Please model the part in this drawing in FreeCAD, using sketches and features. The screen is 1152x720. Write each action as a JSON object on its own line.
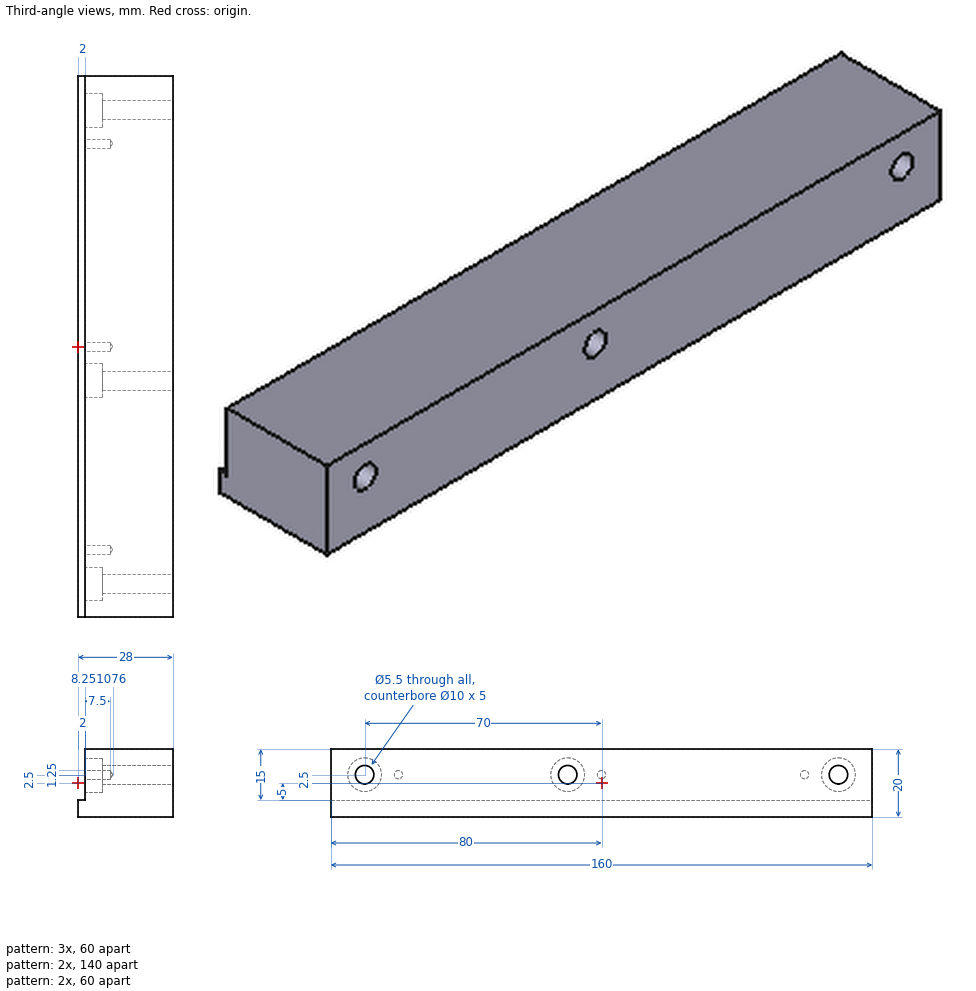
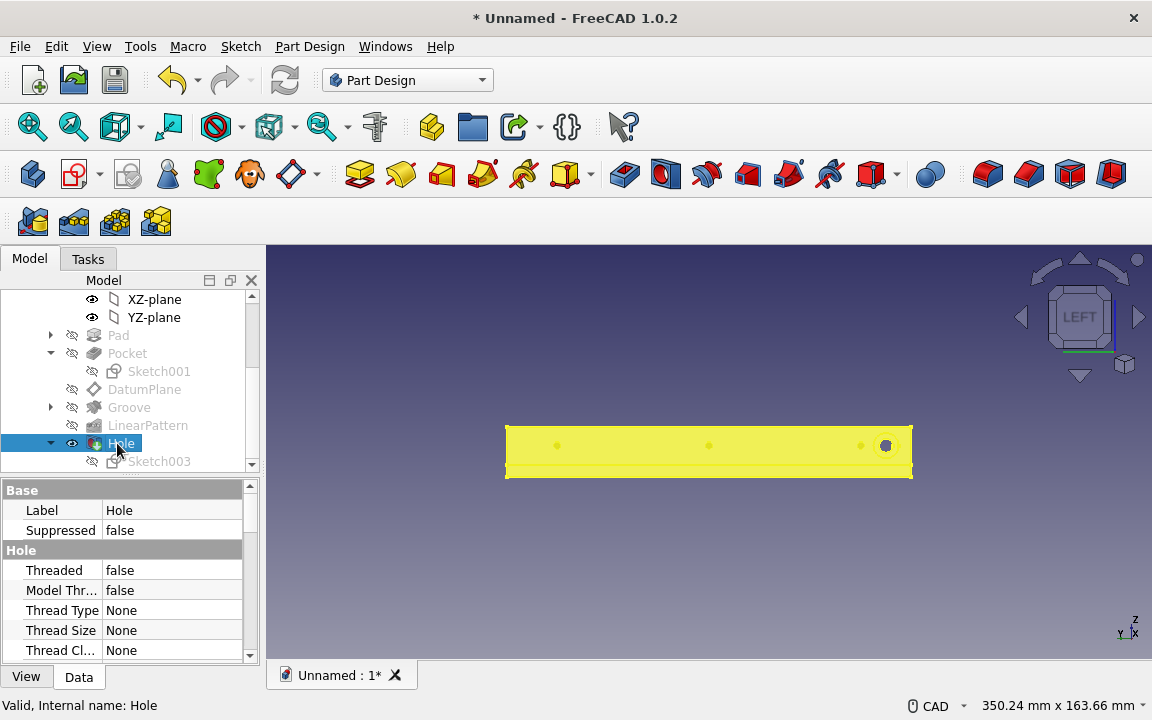
{"action": "left_click", "coordinate": [74, 222]}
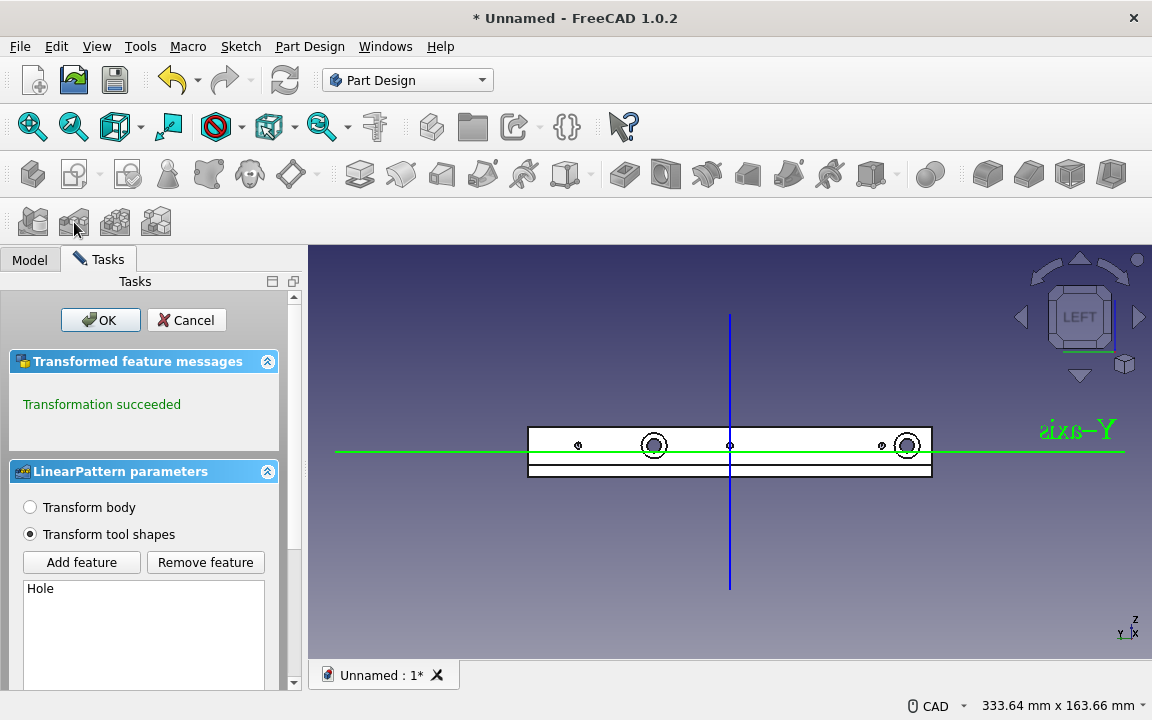
{"action": "scroll", "coordinate": [294, 490], "scroll_direction": "down", "scroll_amount": 2}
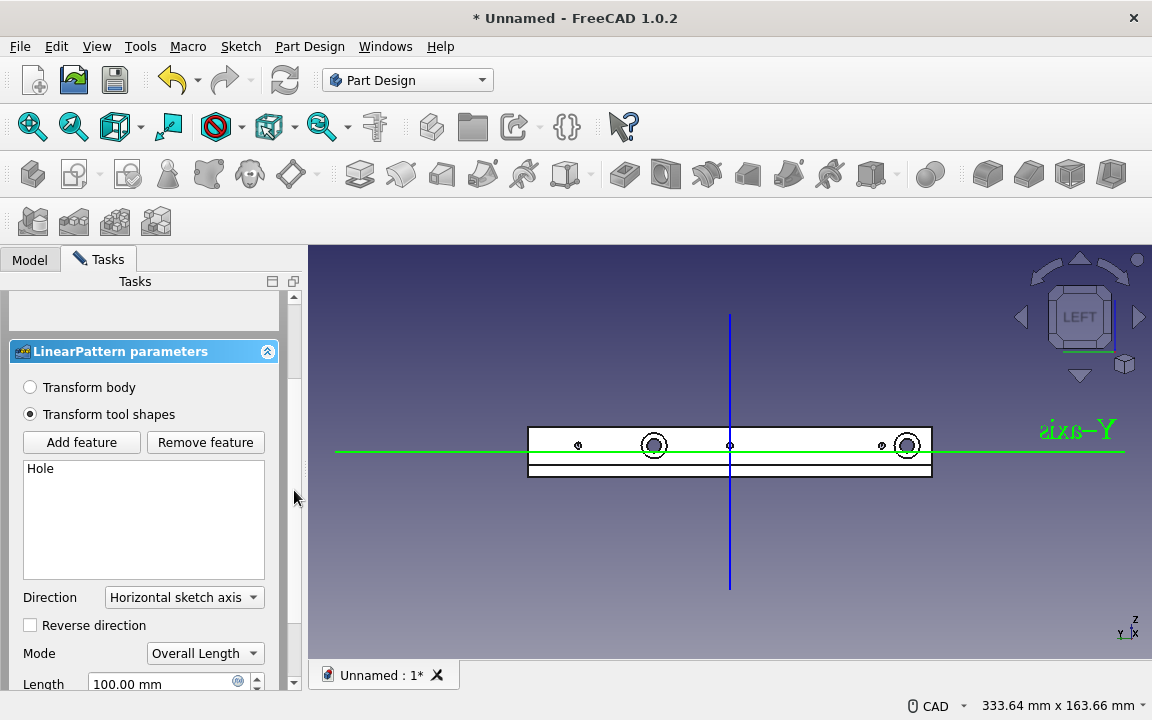
{"action": "left_click", "coordinate": [185, 598]}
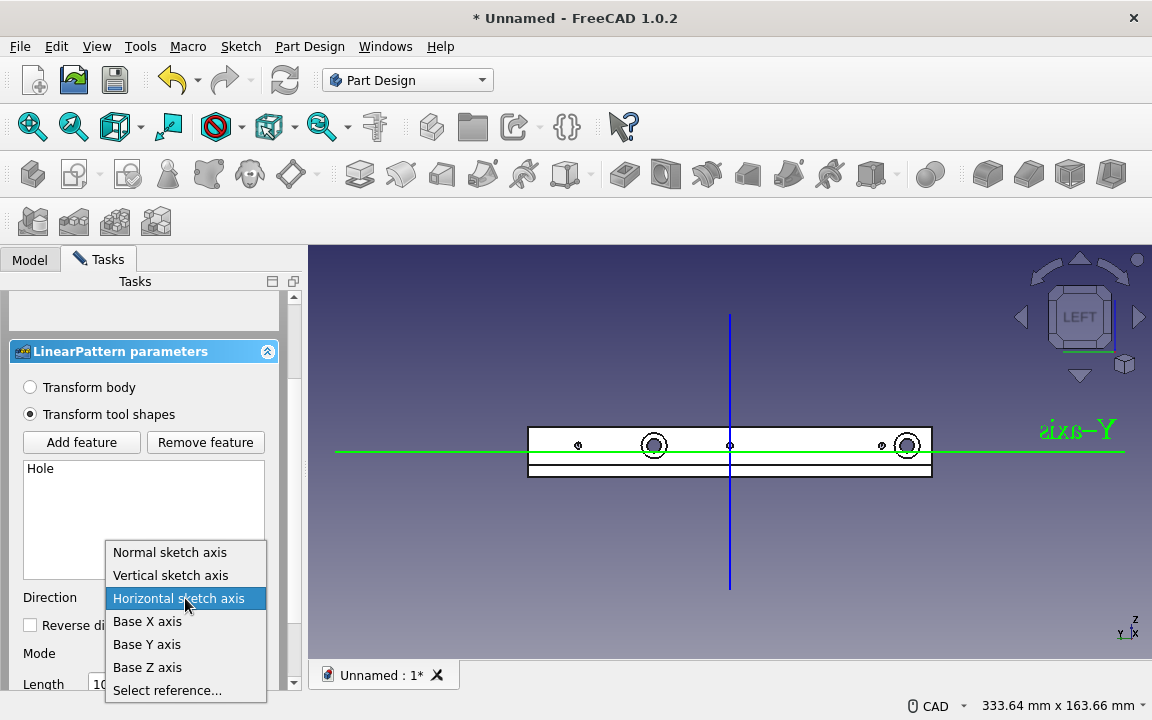
{"action": "left_click", "coordinate": [184, 644]}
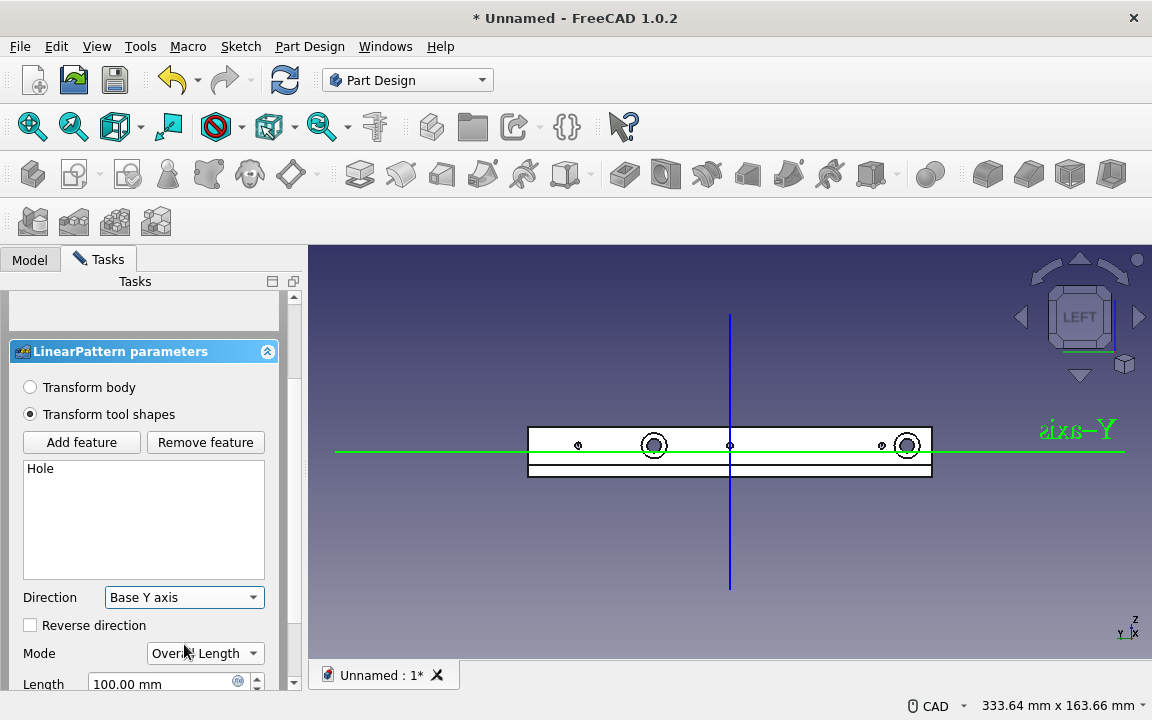
{"action": "left_click", "coordinate": [206, 654]}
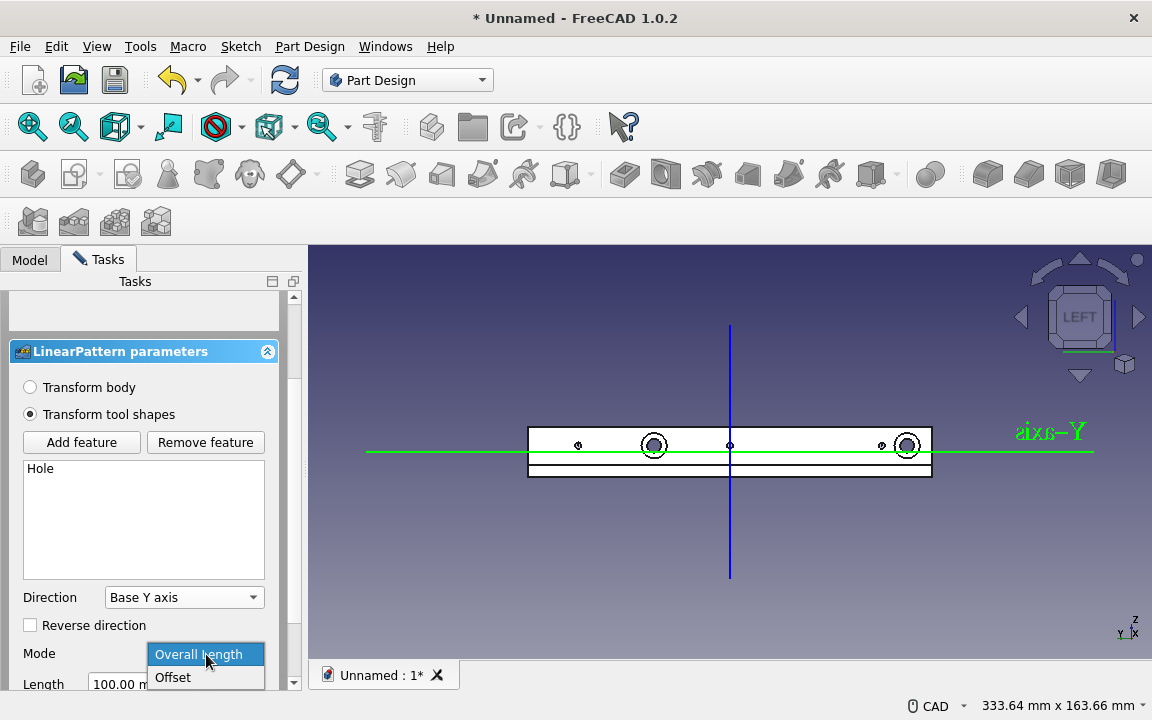
{"action": "left_click", "coordinate": [204, 678]}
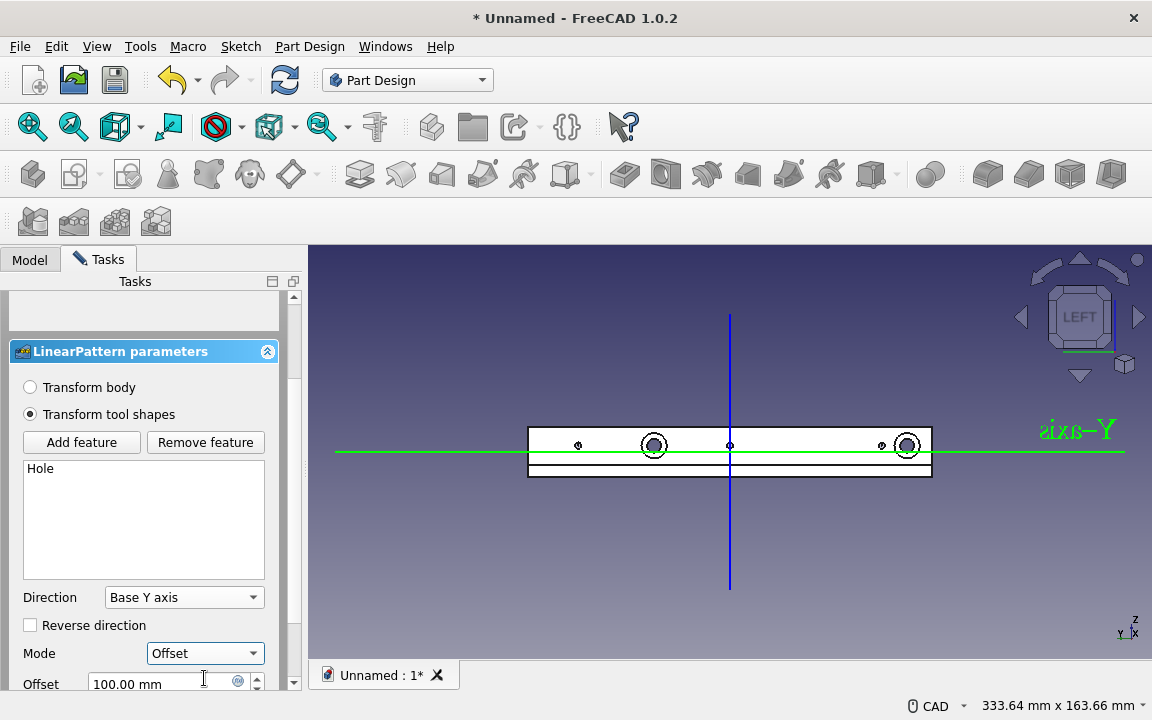
{"action": "scroll", "coordinate": [294, 490], "scroll_direction": "down", "scroll_amount": 2}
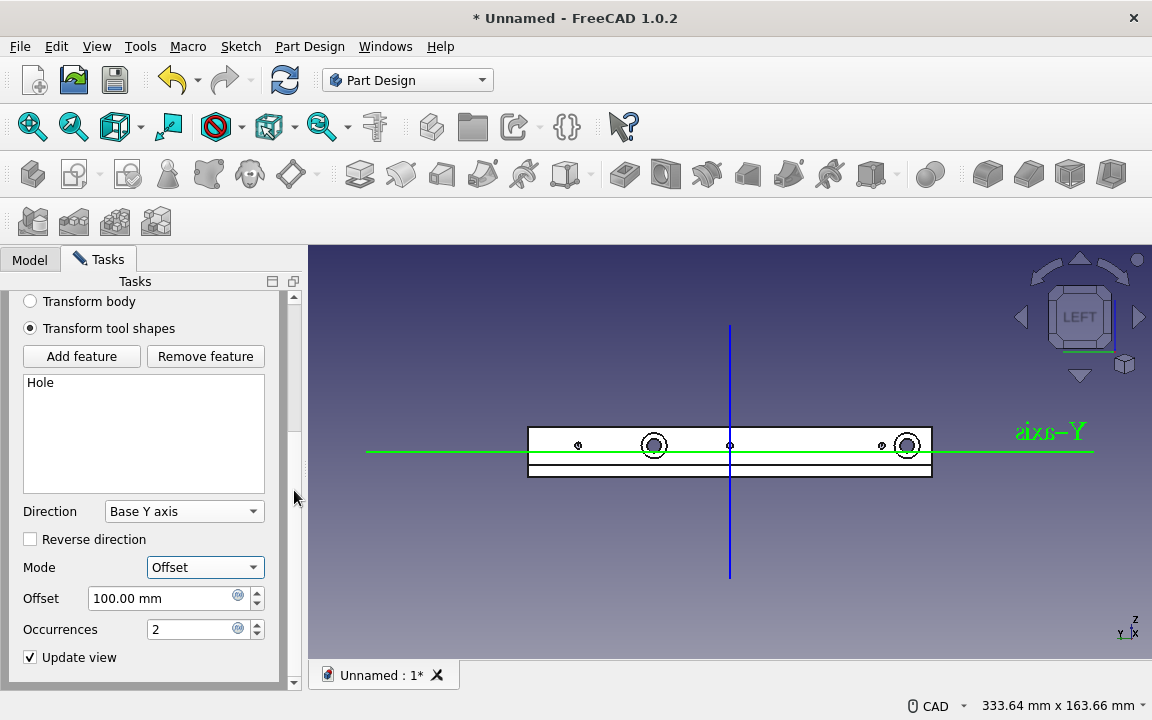
{"action": "triple_click", "coordinate": [170, 598]}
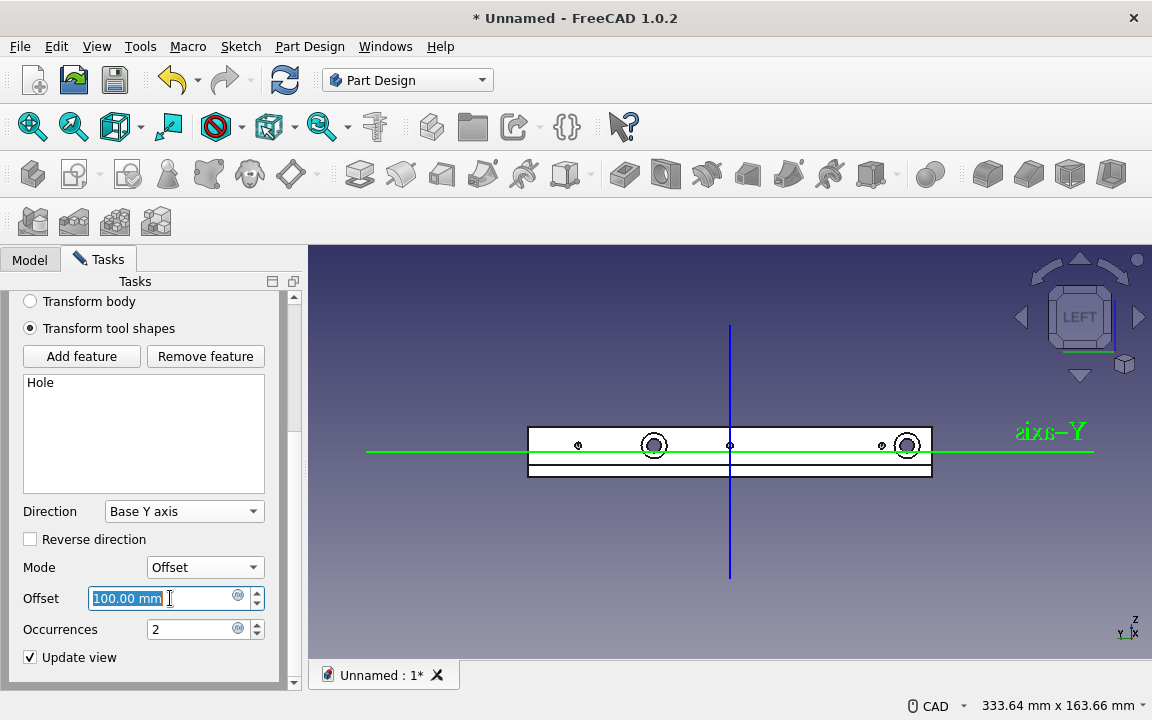
{"action": "type", "text": "140"}
{"action": "key", "text": "Tab"}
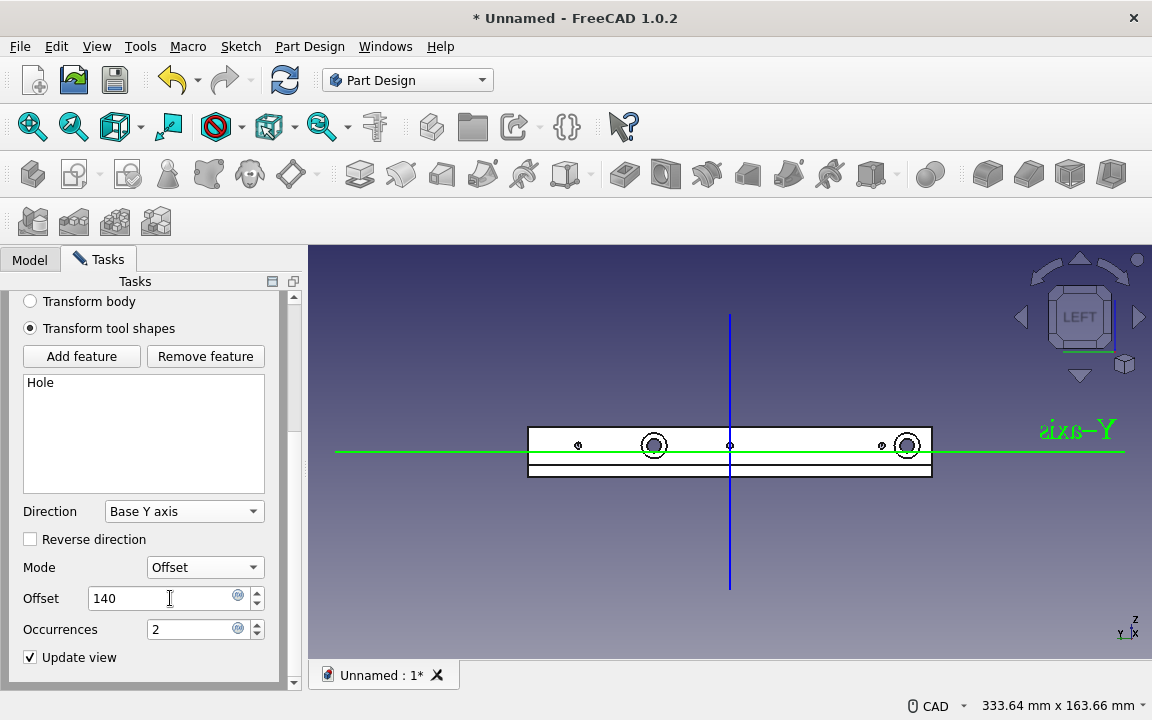
{"action": "triple_click", "coordinate": [199, 630]}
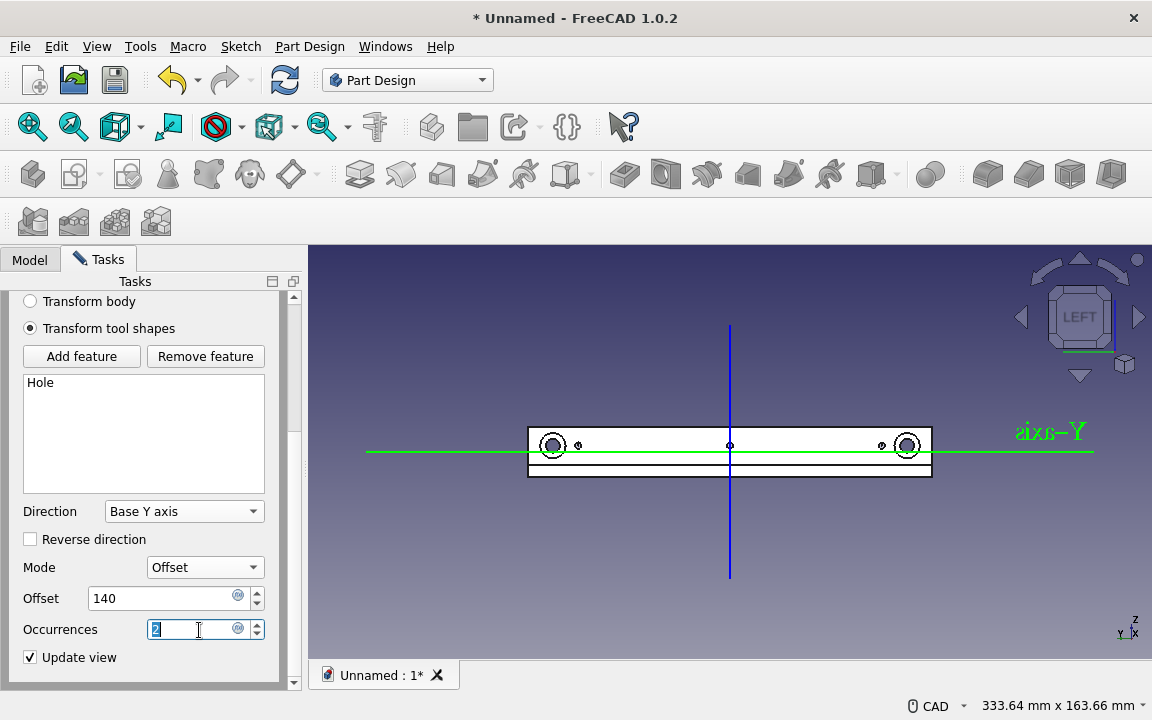
{"action": "type", "text": "2"}
{"action": "key", "text": "Tab"}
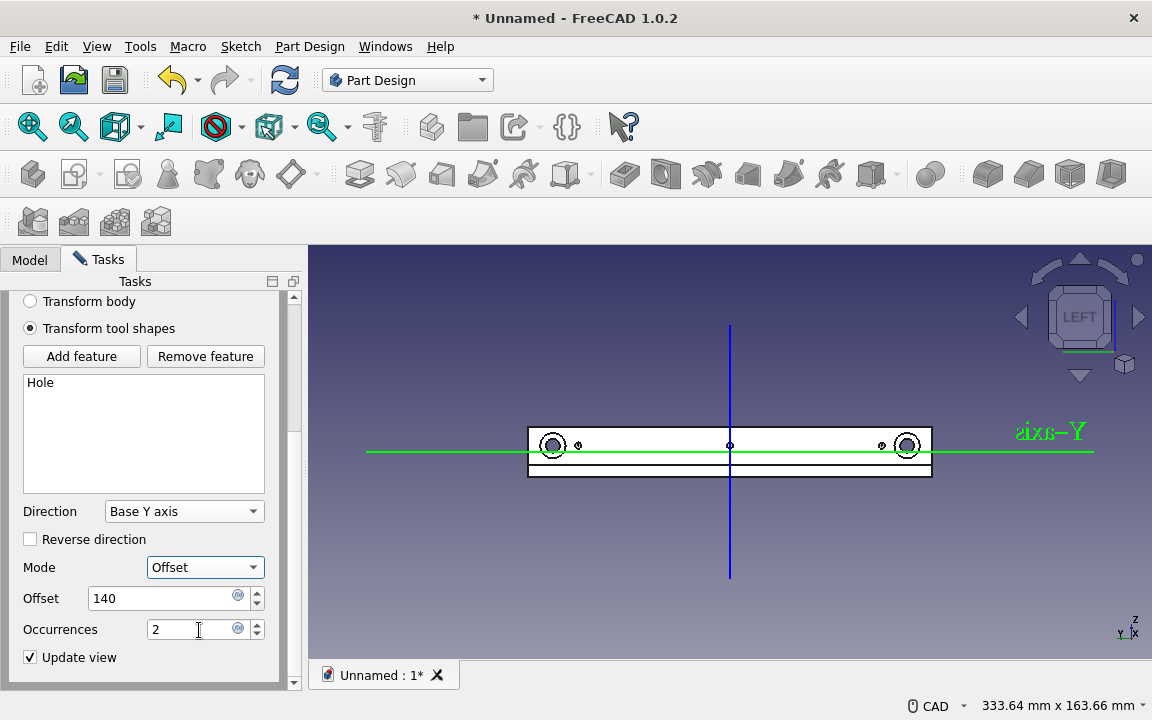
{"action": "scroll", "coordinate": [294, 490], "scroll_direction": "up", "scroll_amount": 5}